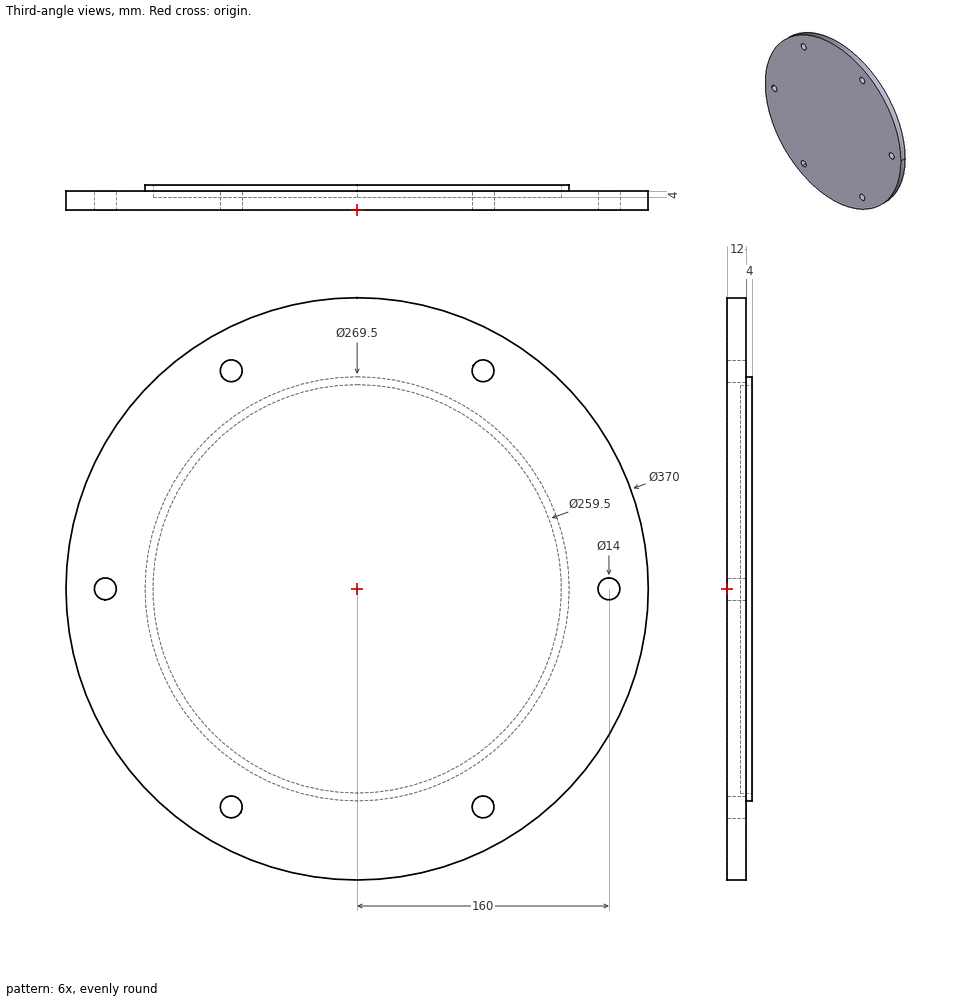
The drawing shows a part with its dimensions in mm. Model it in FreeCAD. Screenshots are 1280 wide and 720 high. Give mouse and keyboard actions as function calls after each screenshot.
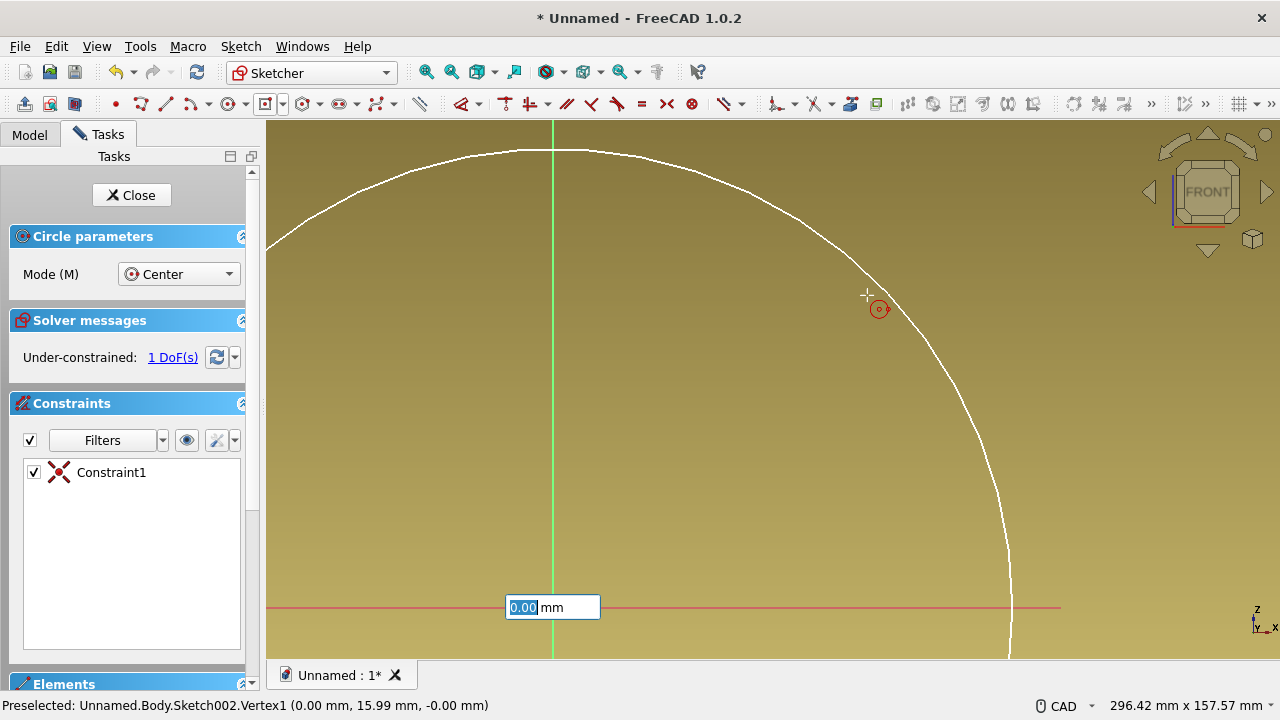
click(867, 294)
key(Escape)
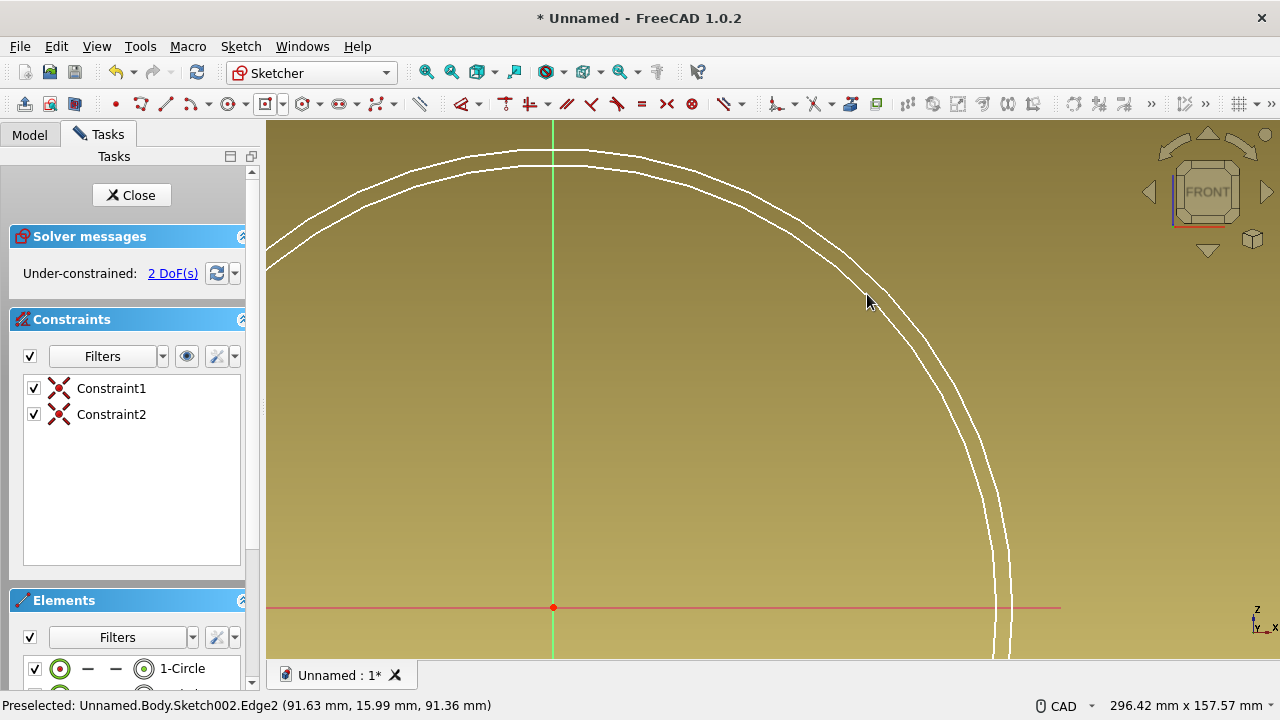
click(460, 104)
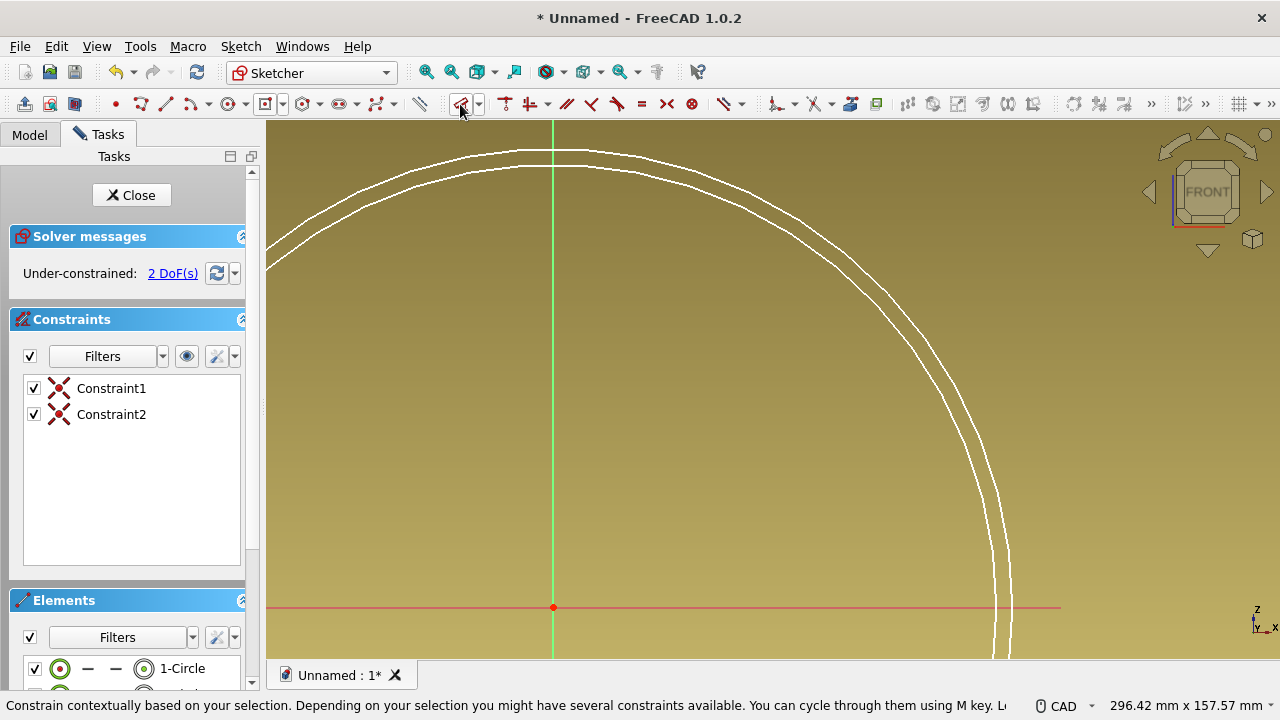
click(877, 282)
click(900, 259)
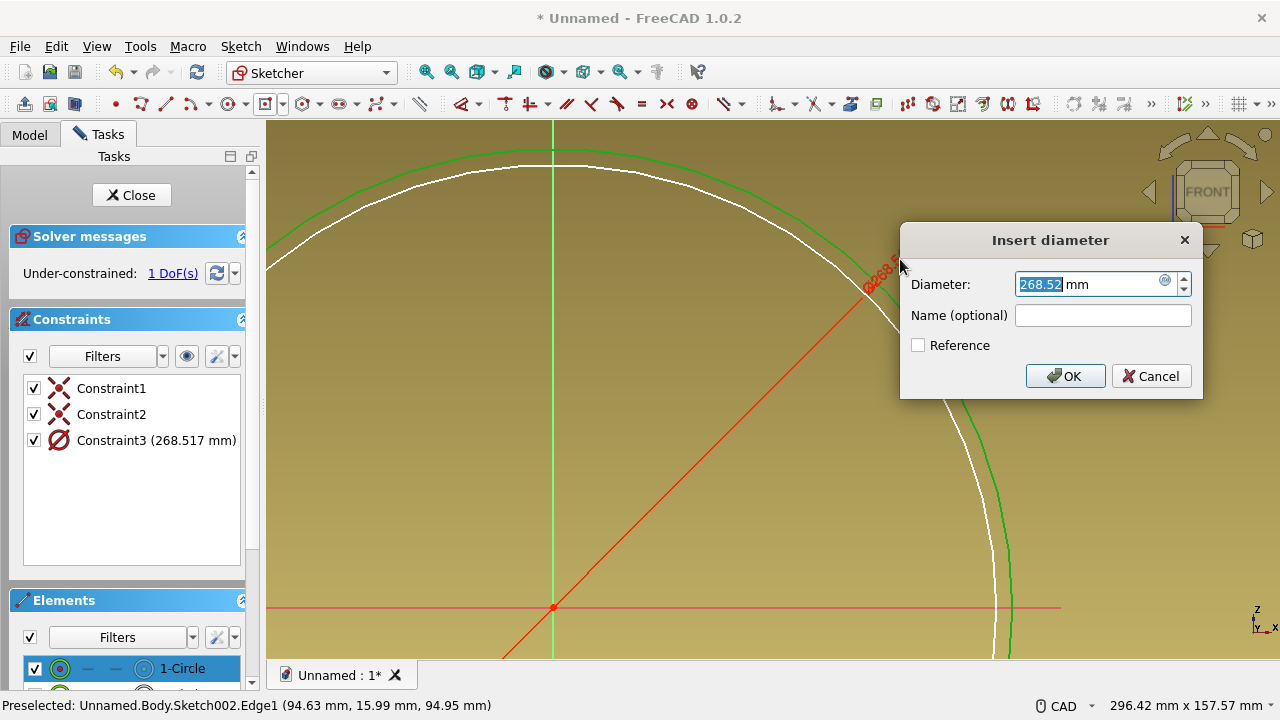
text(269.5)
key(Return)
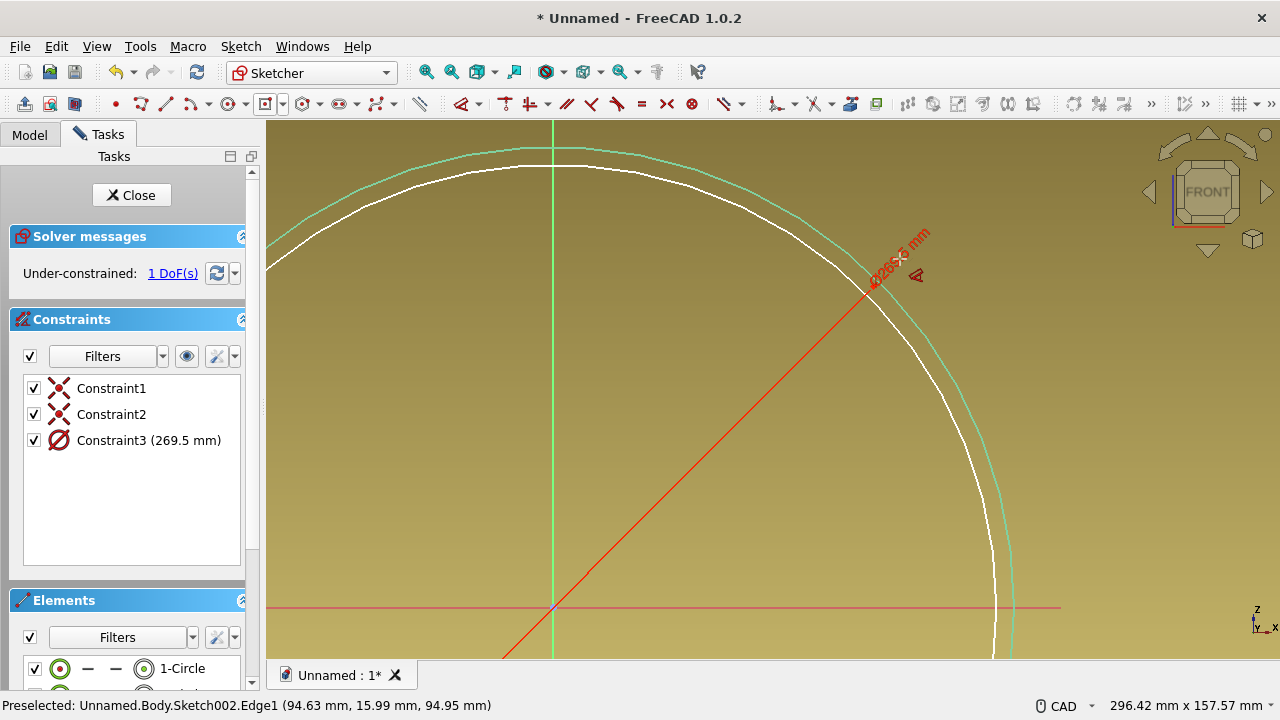
click(866, 294)
click(1009, 473)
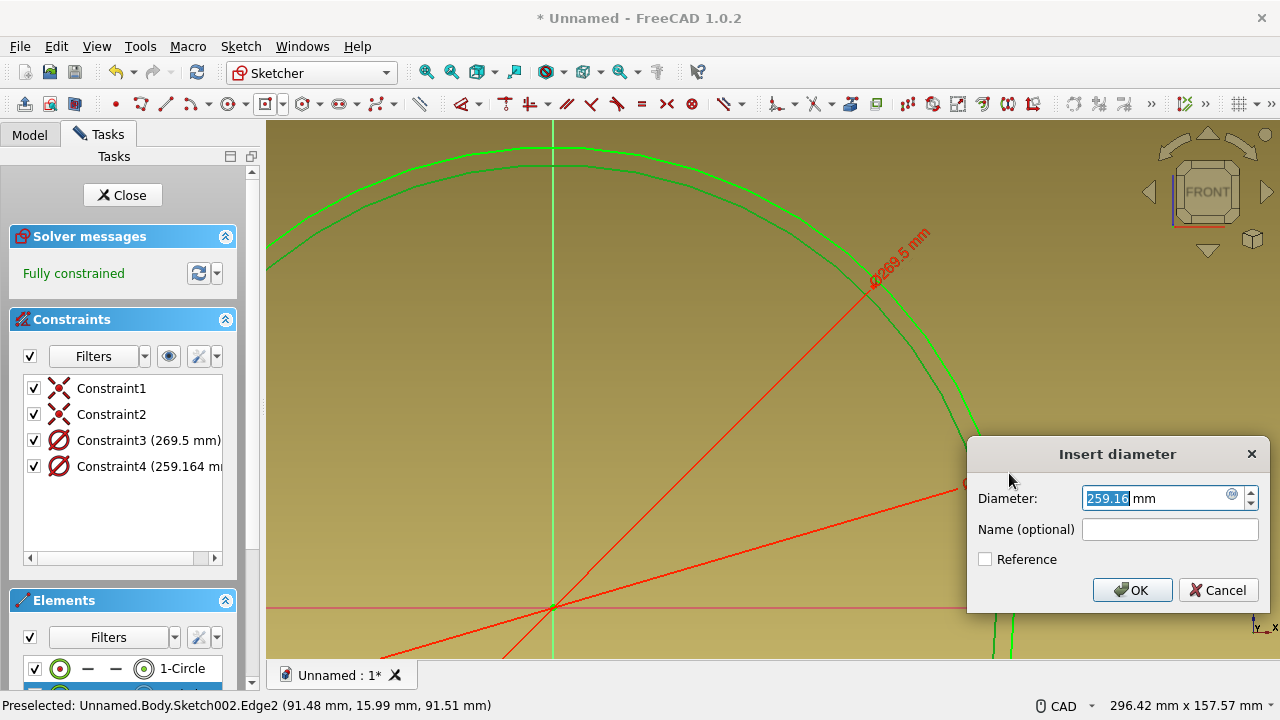
text(259.5)
key(Return)
key(Escape)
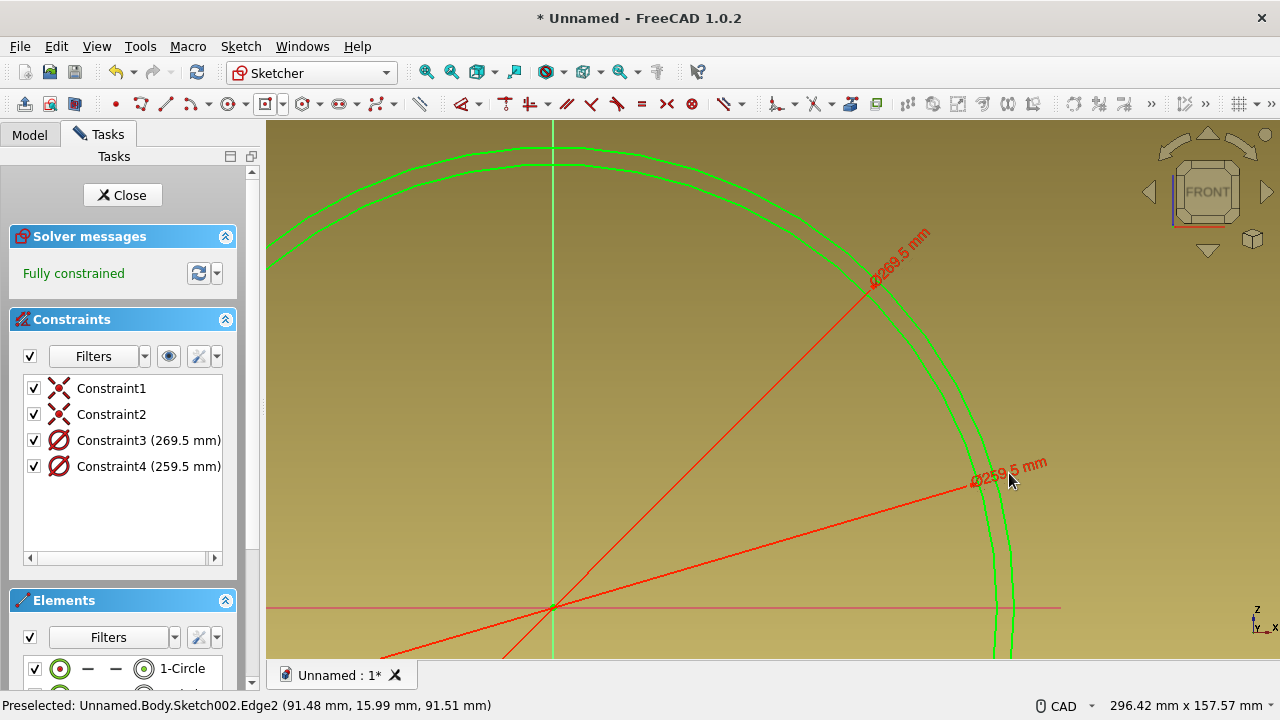
click(123, 195)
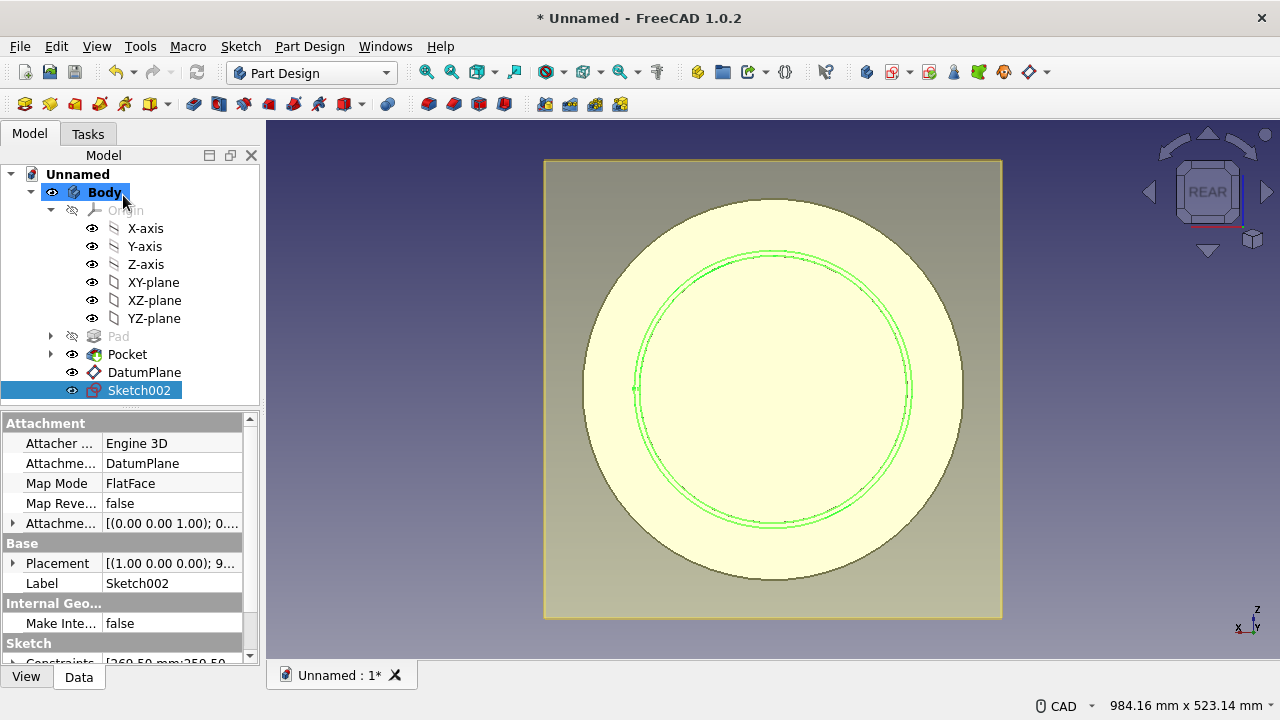
click(25, 104)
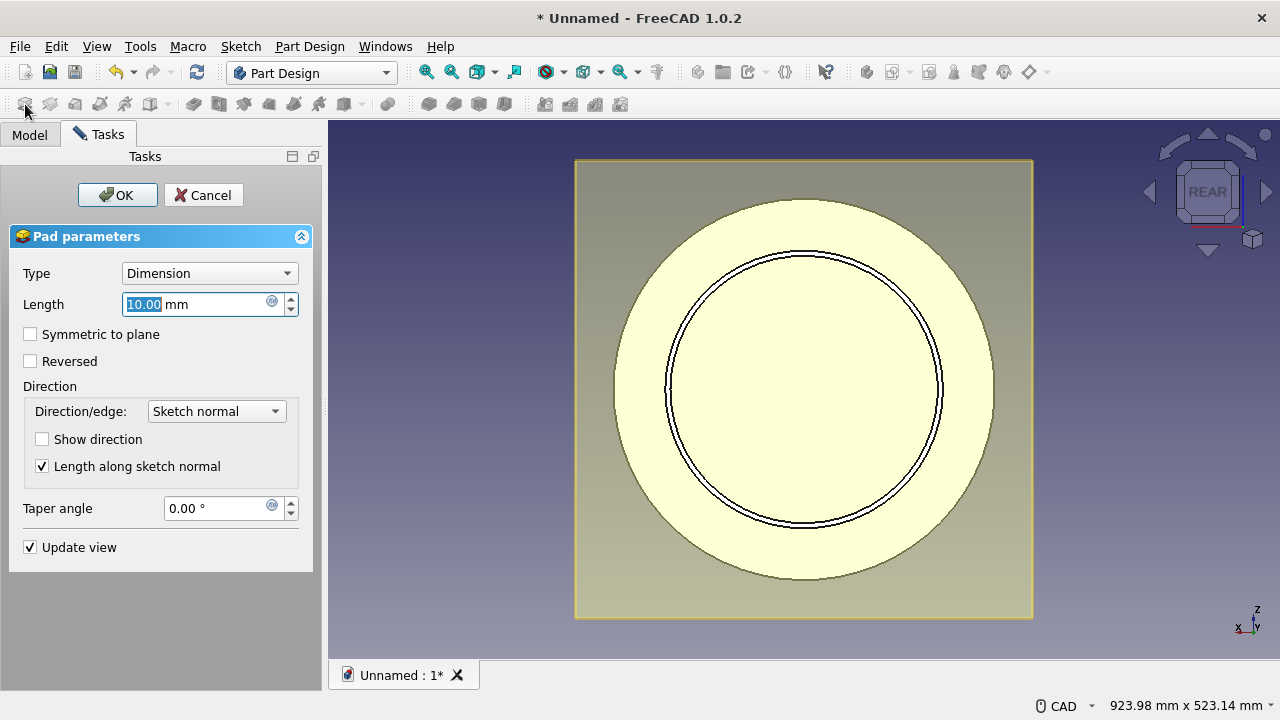
text(4)
key(Tab)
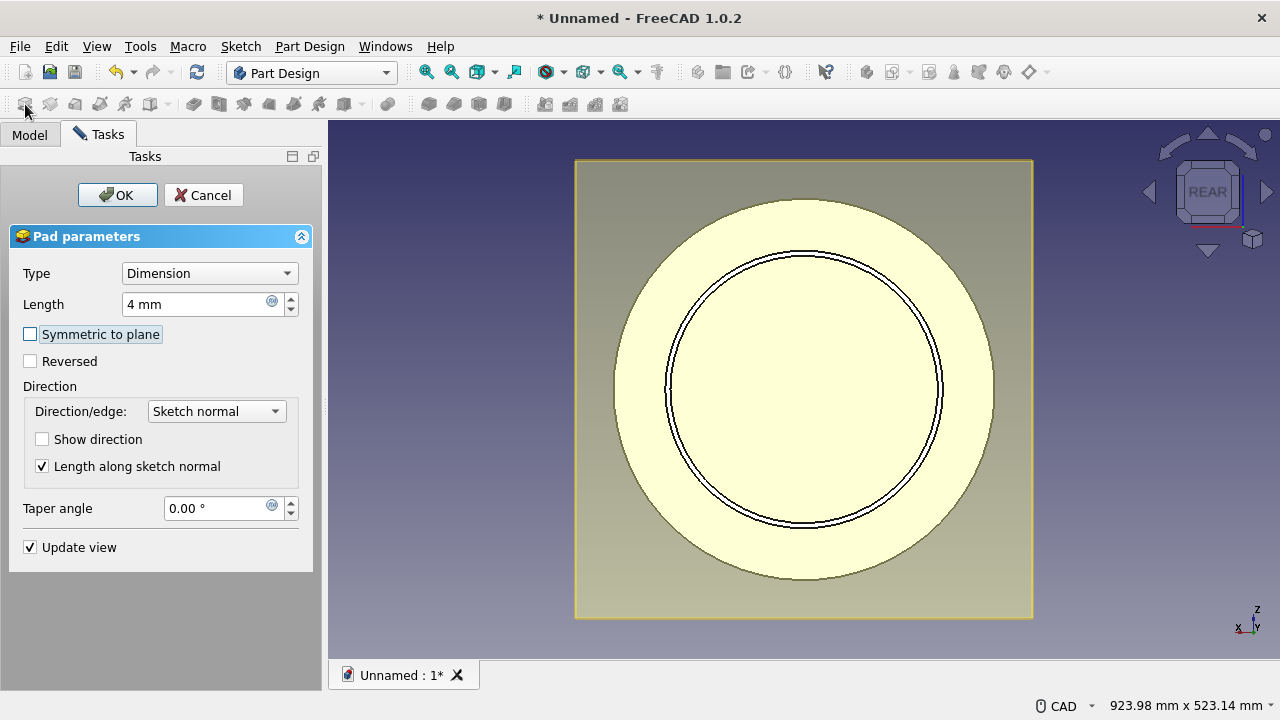
click(118, 195)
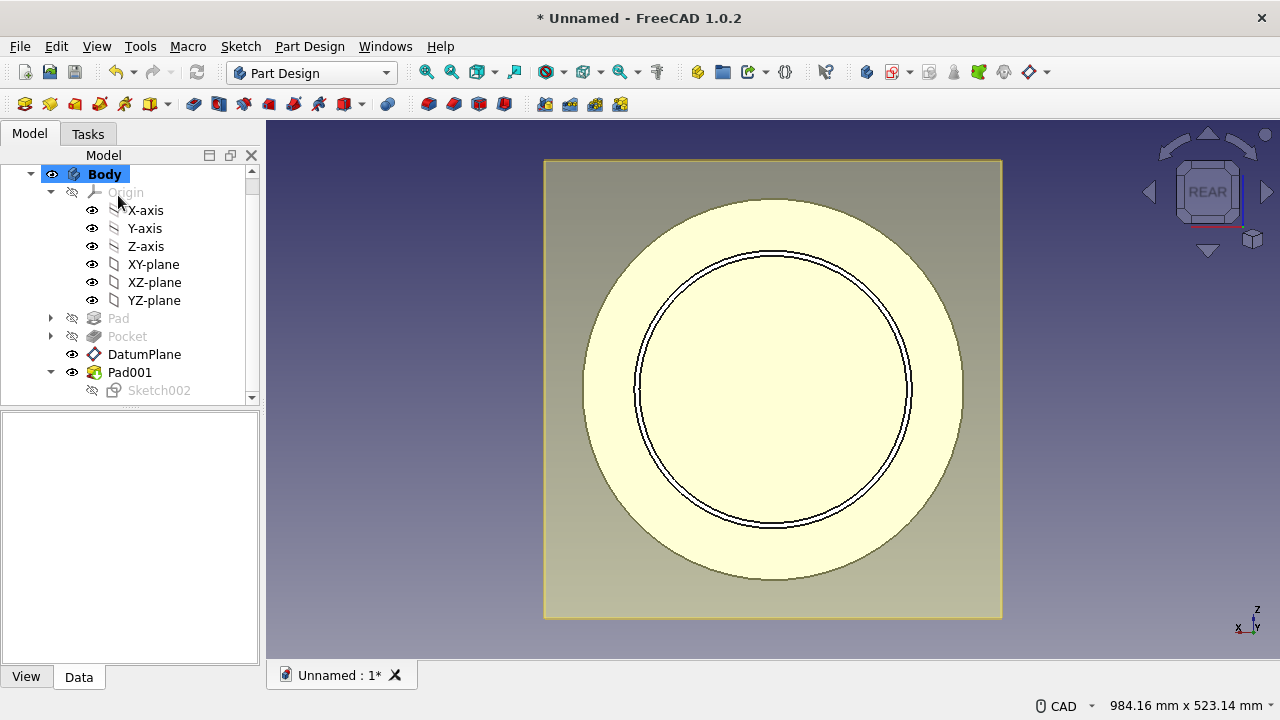
click(117, 354)
key(space)